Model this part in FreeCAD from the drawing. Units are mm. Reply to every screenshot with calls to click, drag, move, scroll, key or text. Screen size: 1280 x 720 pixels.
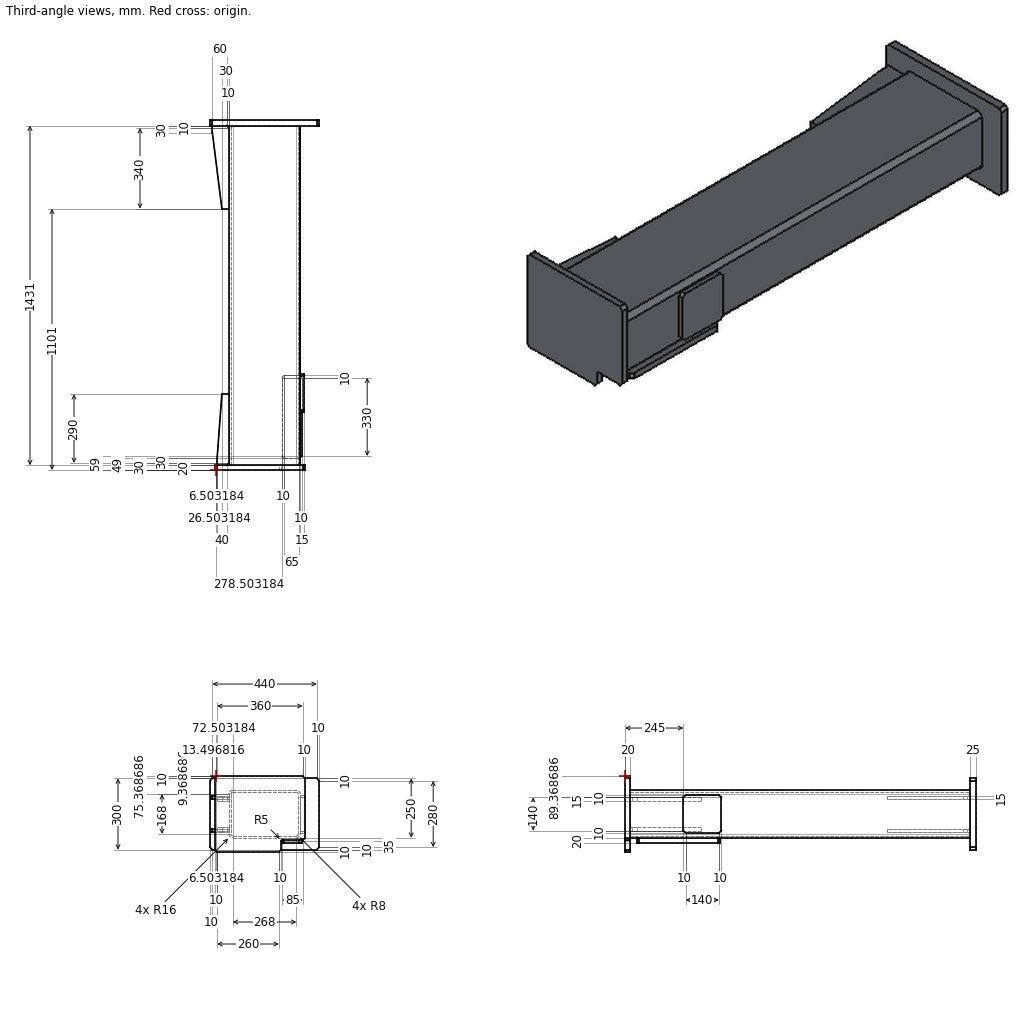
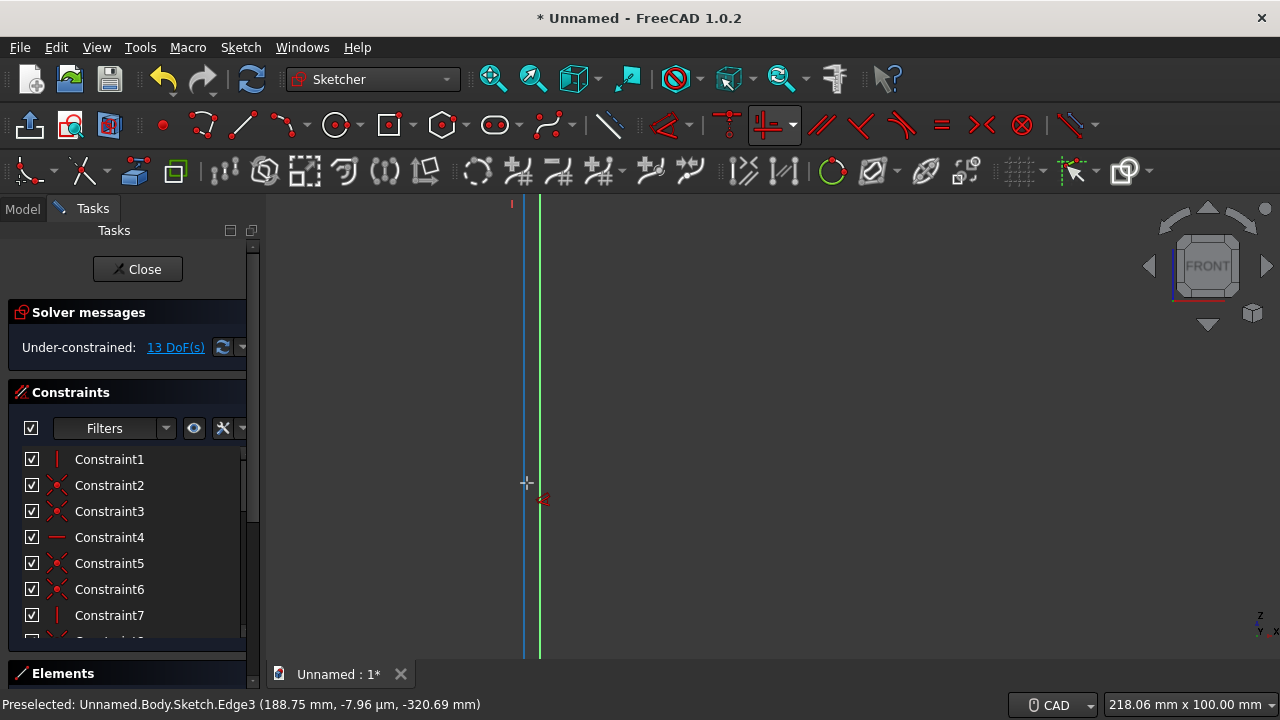
click(524, 482)
click(490, 426)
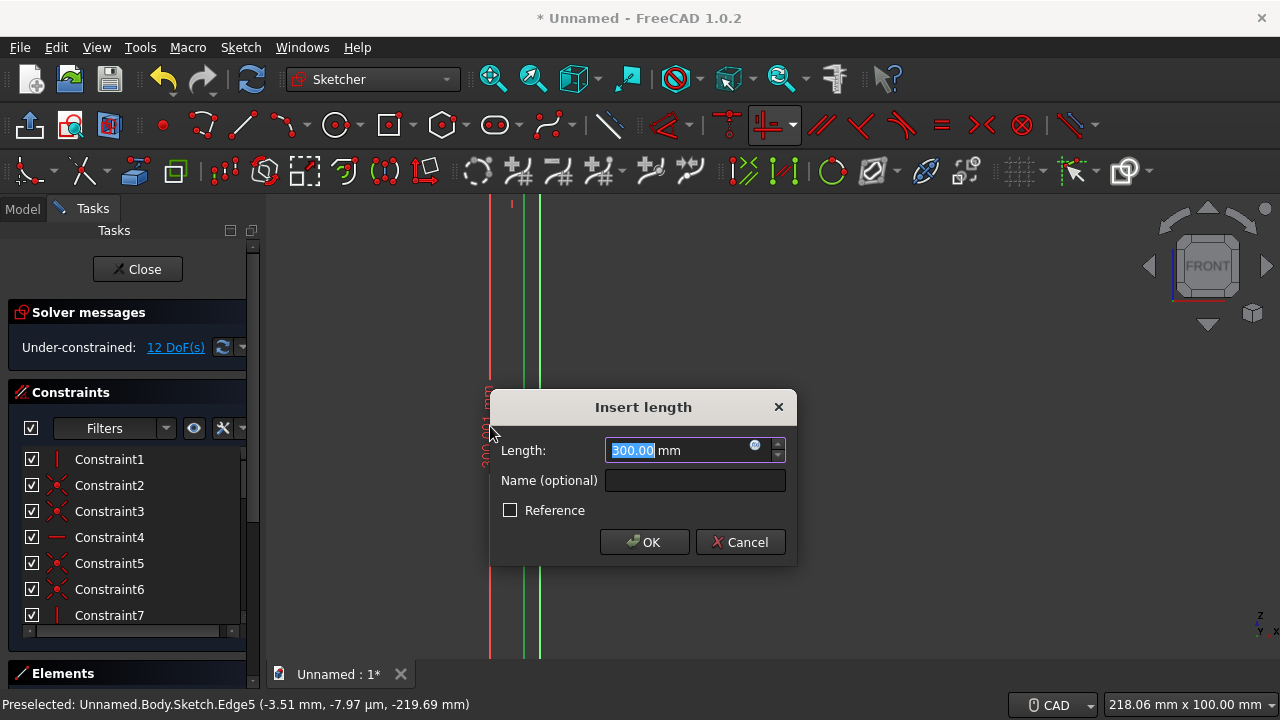
text(300)
key(Return)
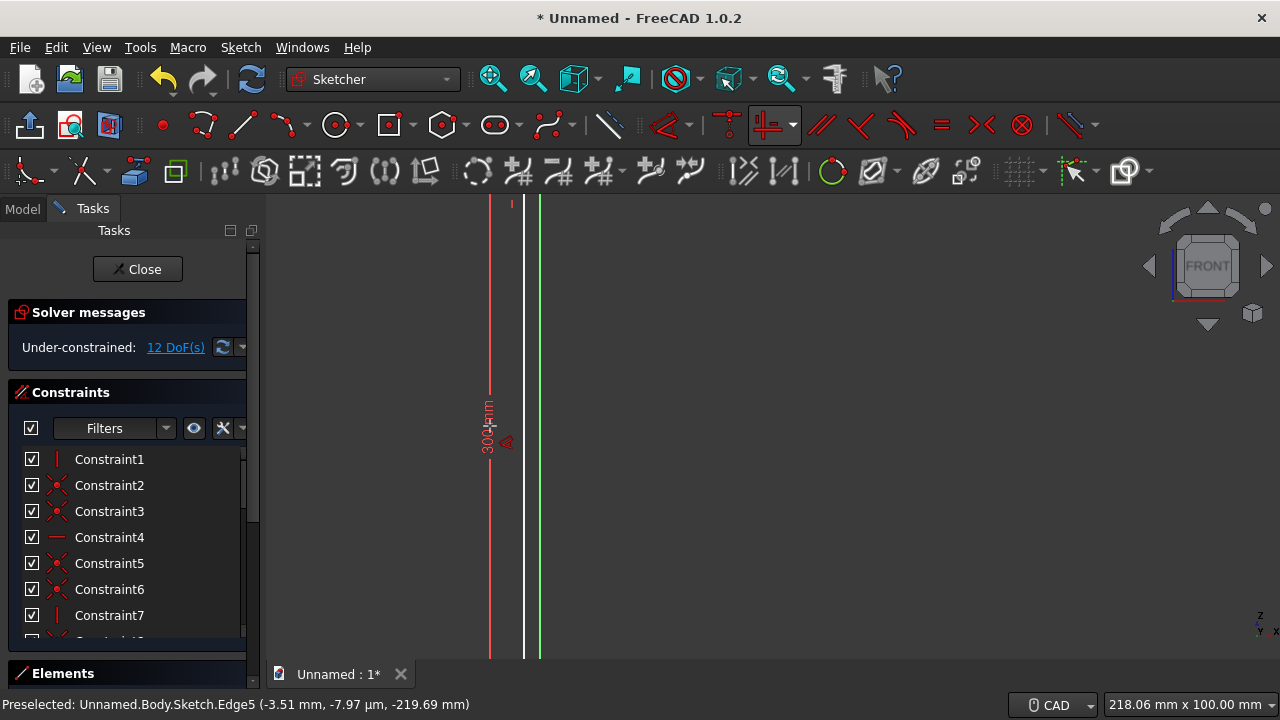
scroll(527, 483, down, 8)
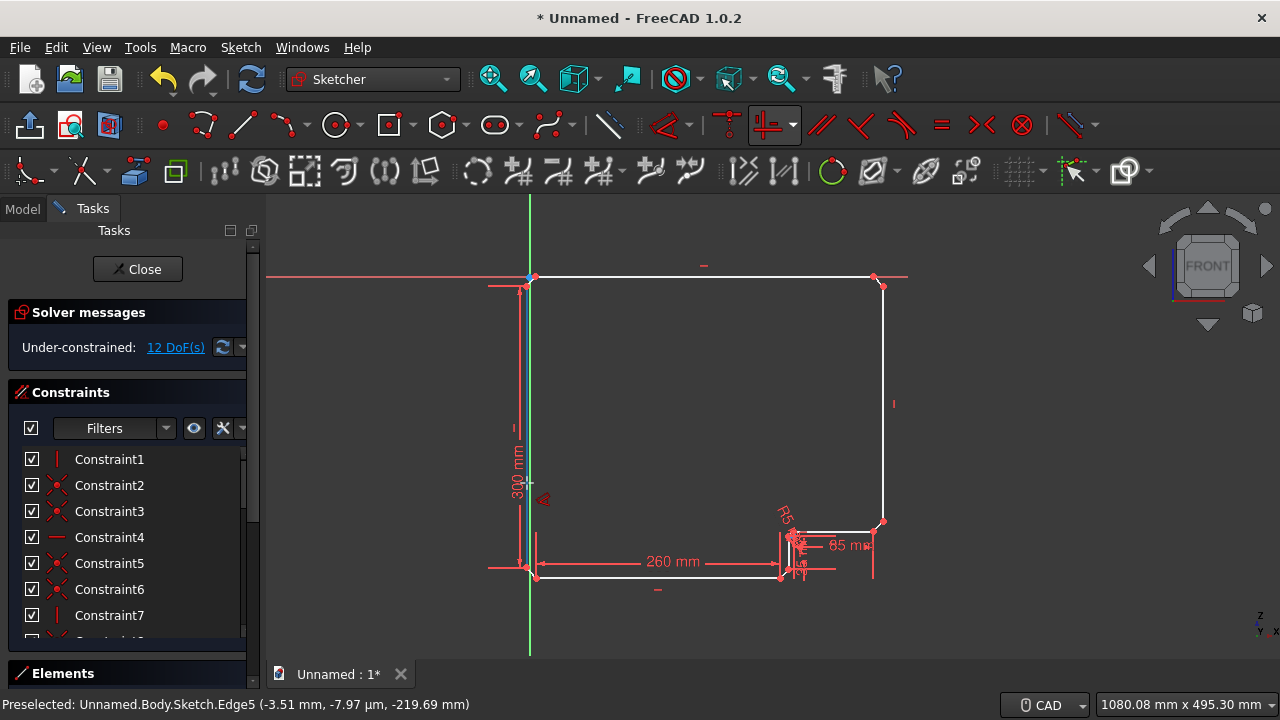
click(637, 277)
click(705, 243)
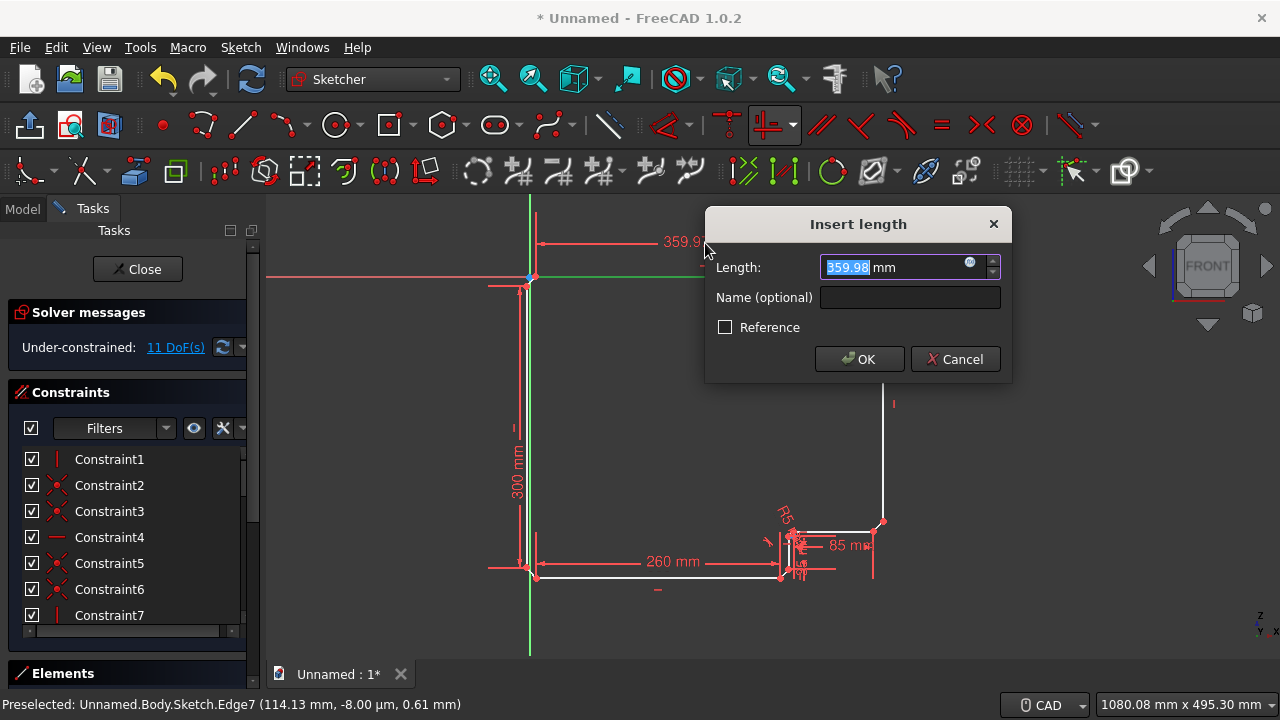
text(360)
key(Return)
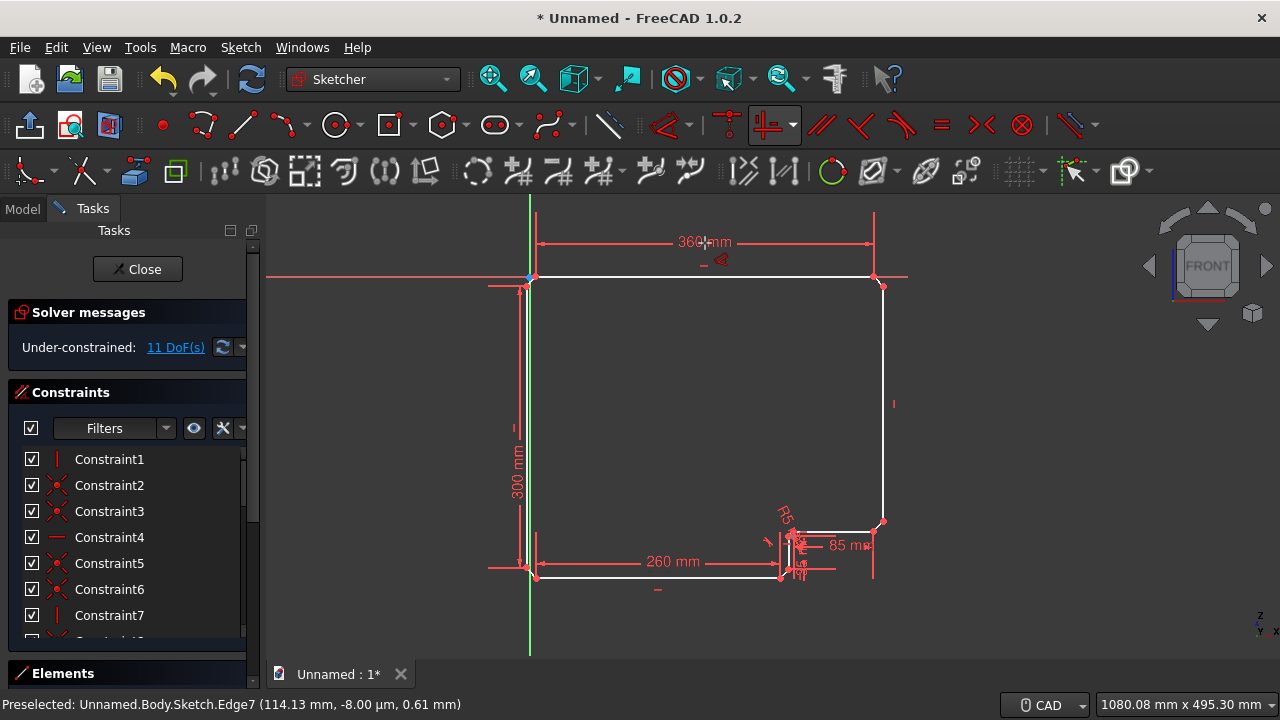
click(883, 357)
click(917, 404)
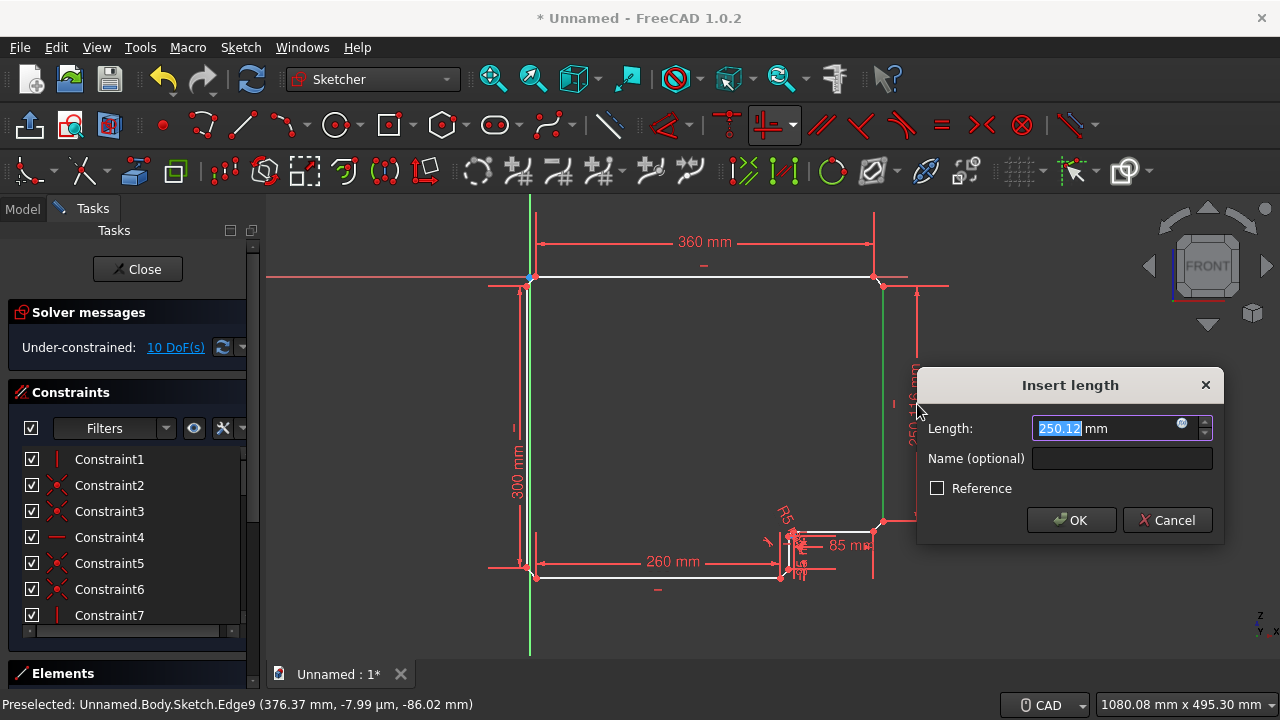
text(250)
key(Return)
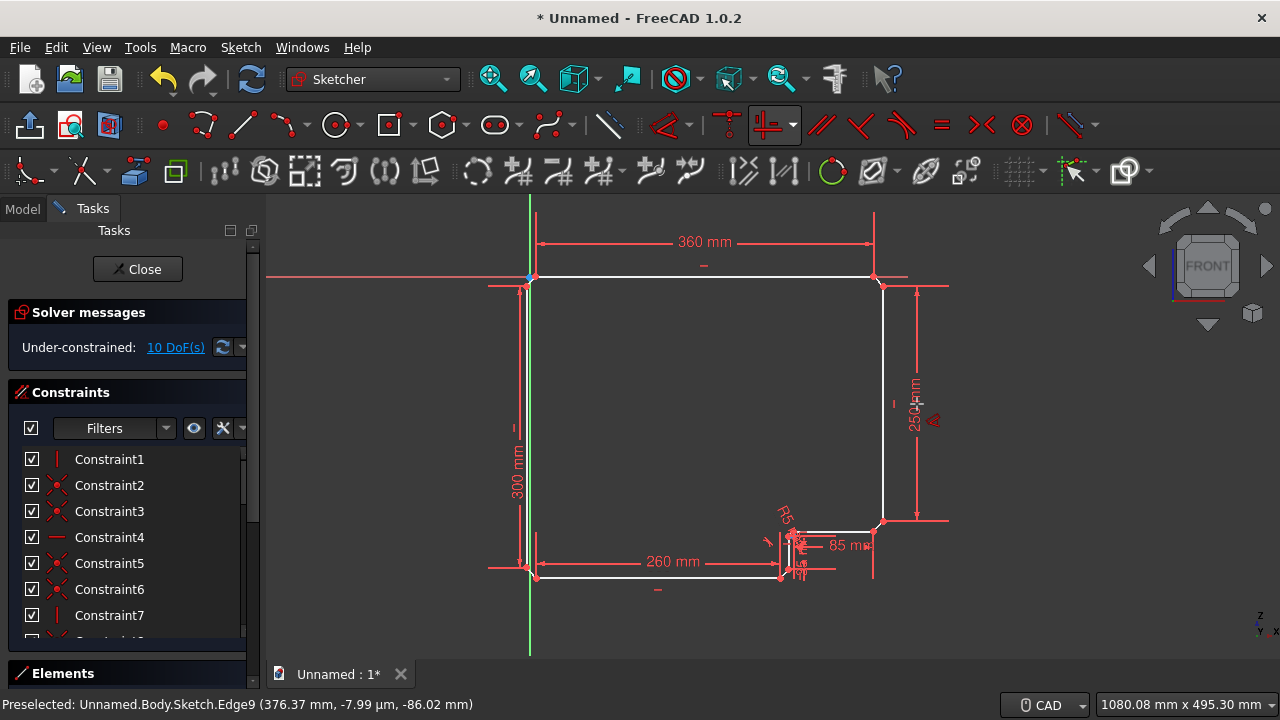
scroll(785, 574, up, 8)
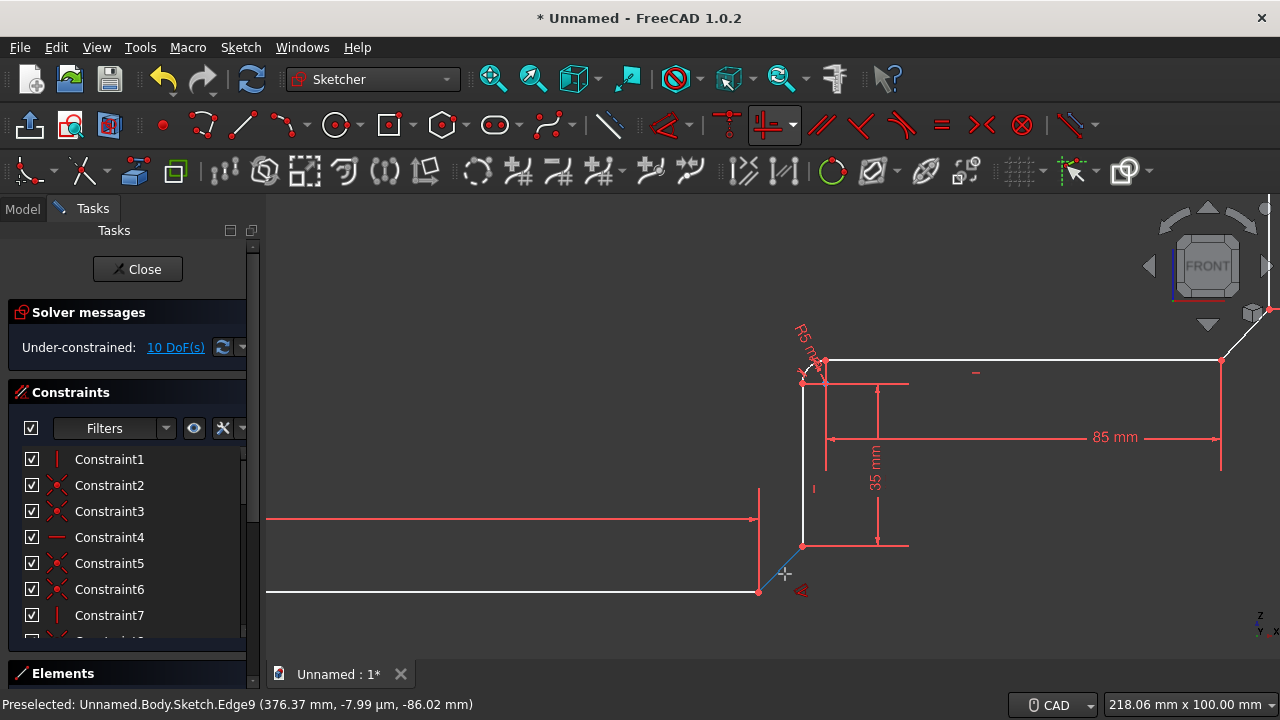
click(781, 569)
click(781, 626)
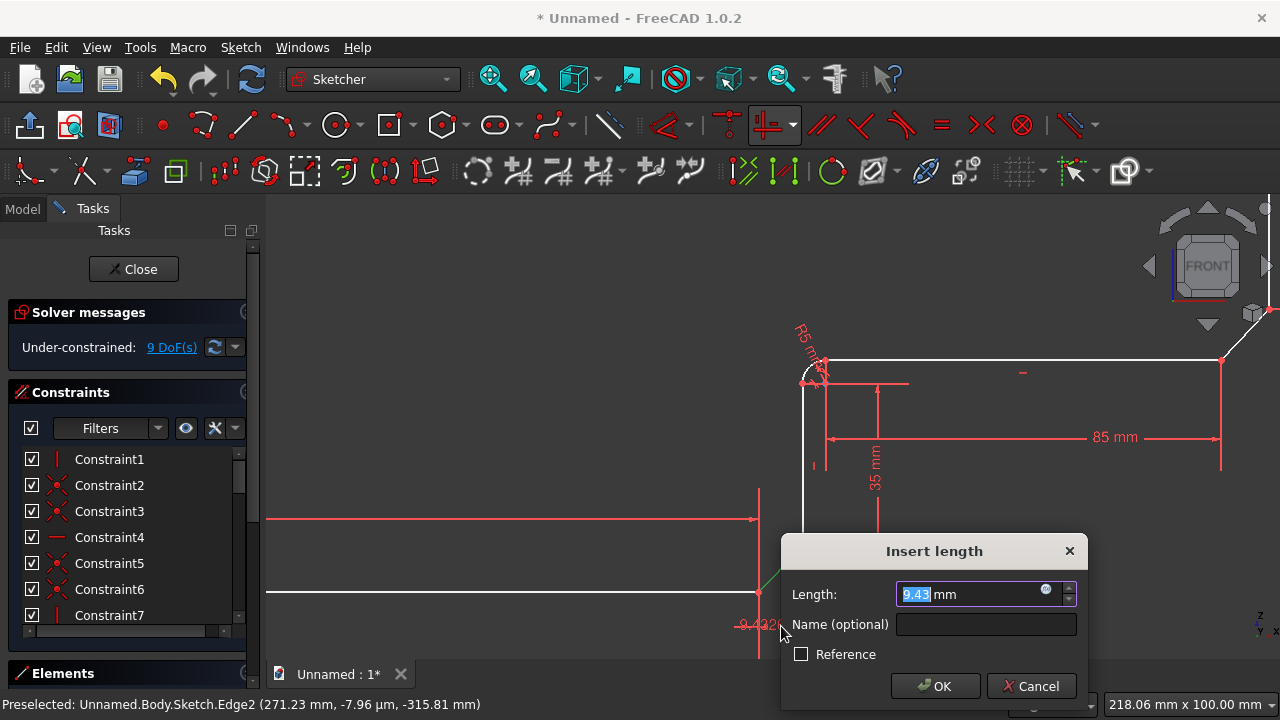
text(10)
key(Return)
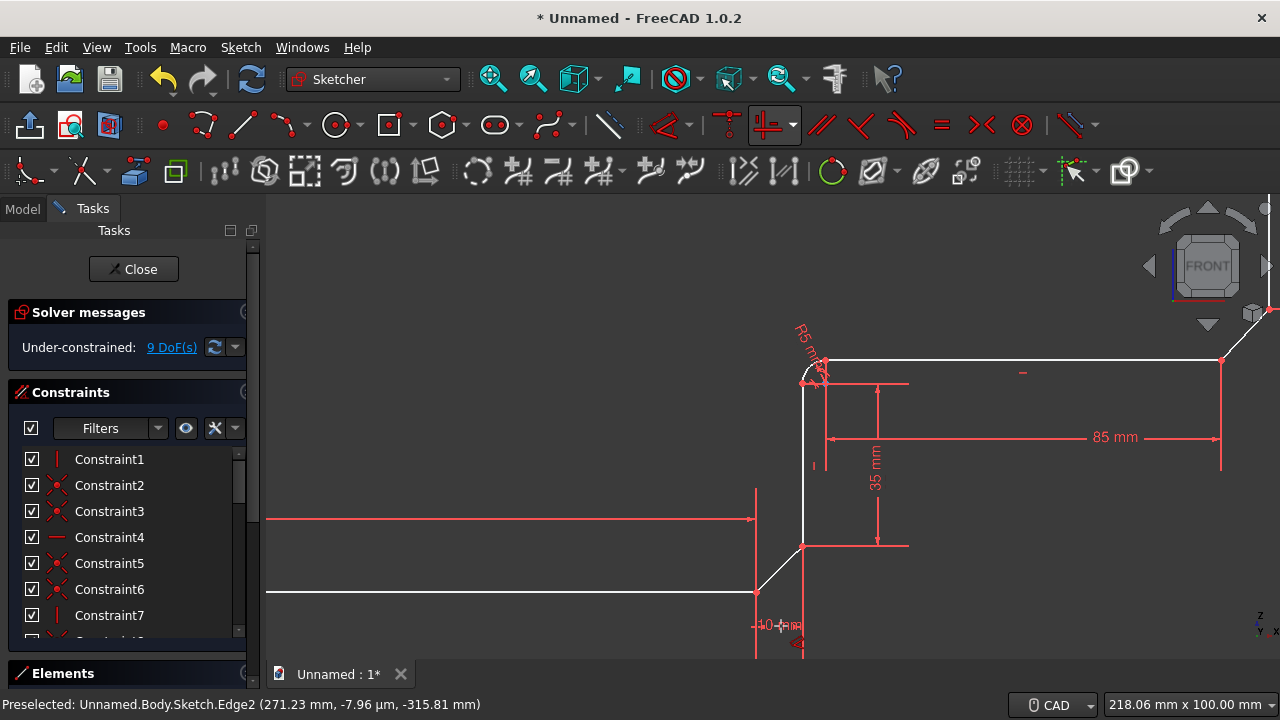
click(789, 560)
click(837, 569)